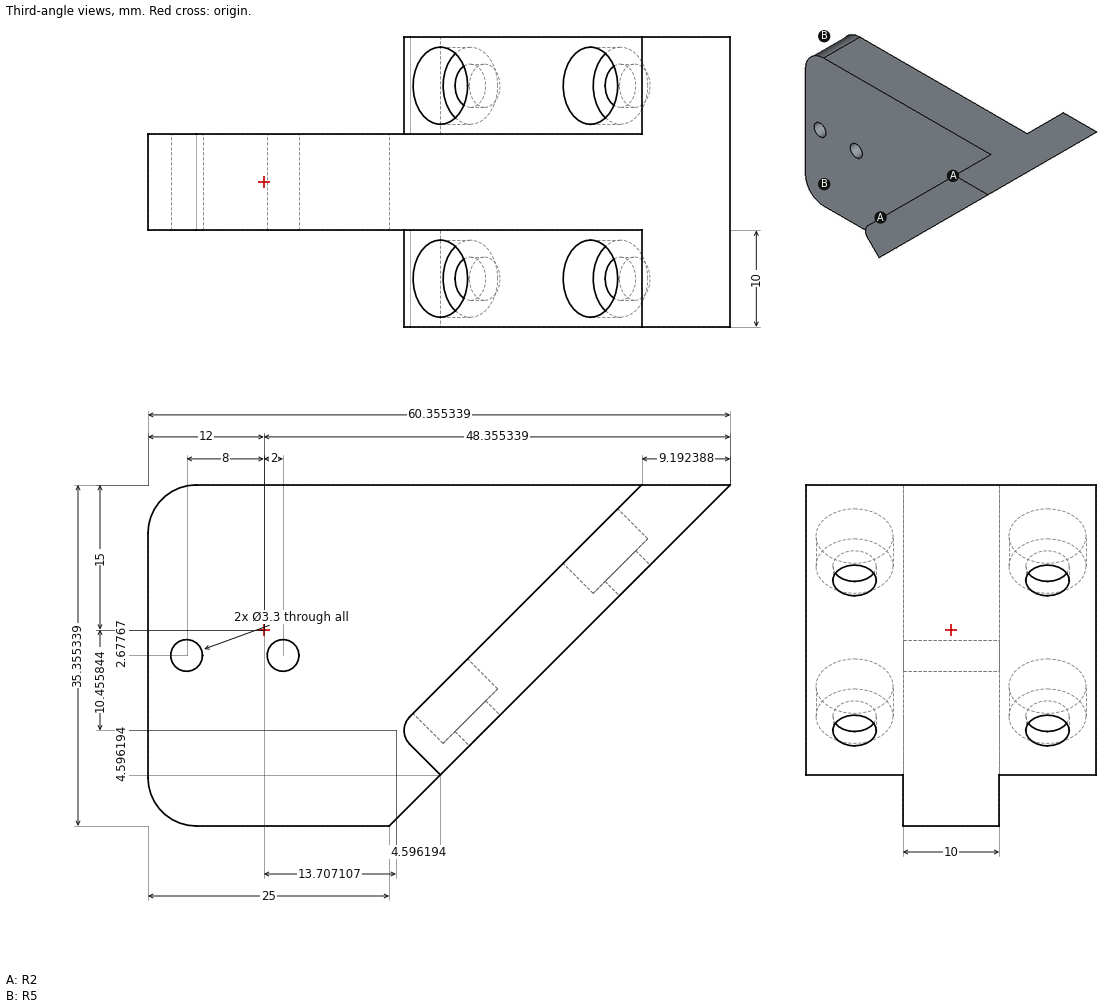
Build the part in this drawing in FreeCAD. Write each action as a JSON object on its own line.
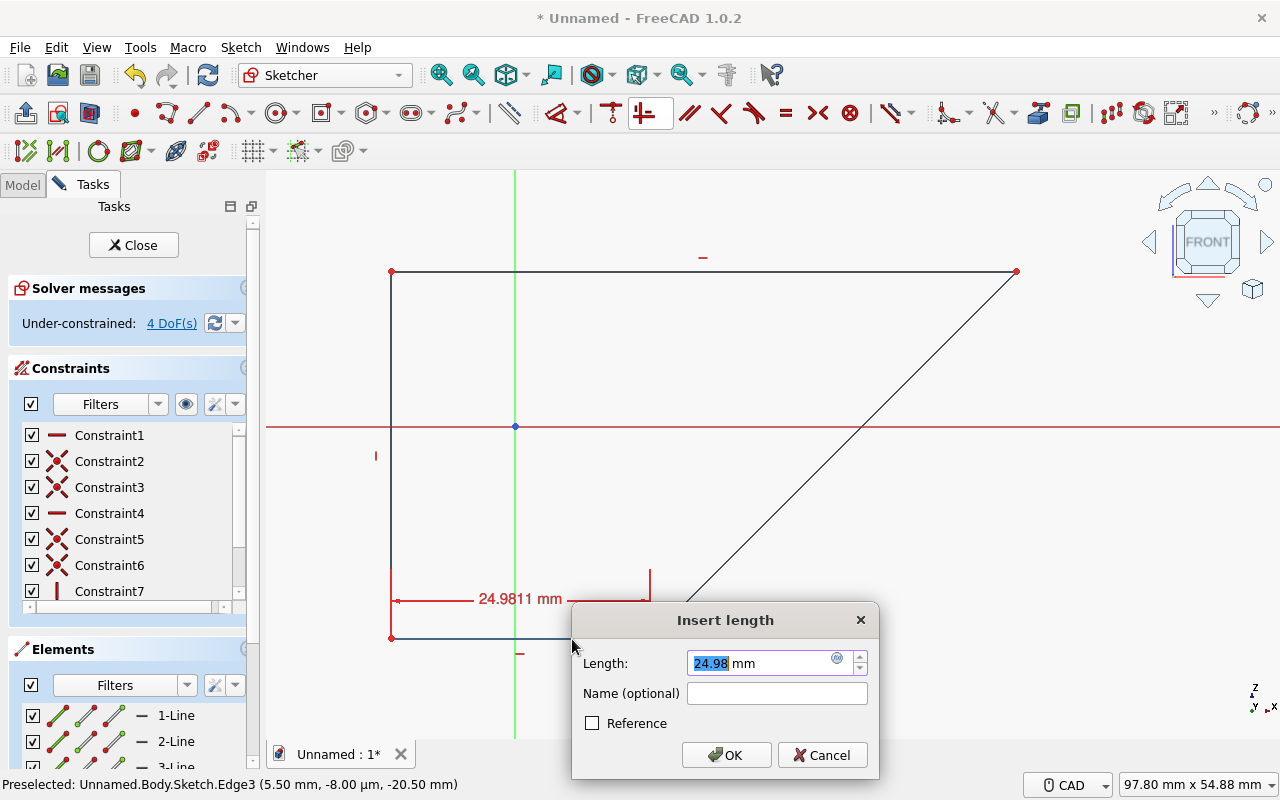
{"action": "type", "text": "25"}
{"action": "key", "text": "Return"}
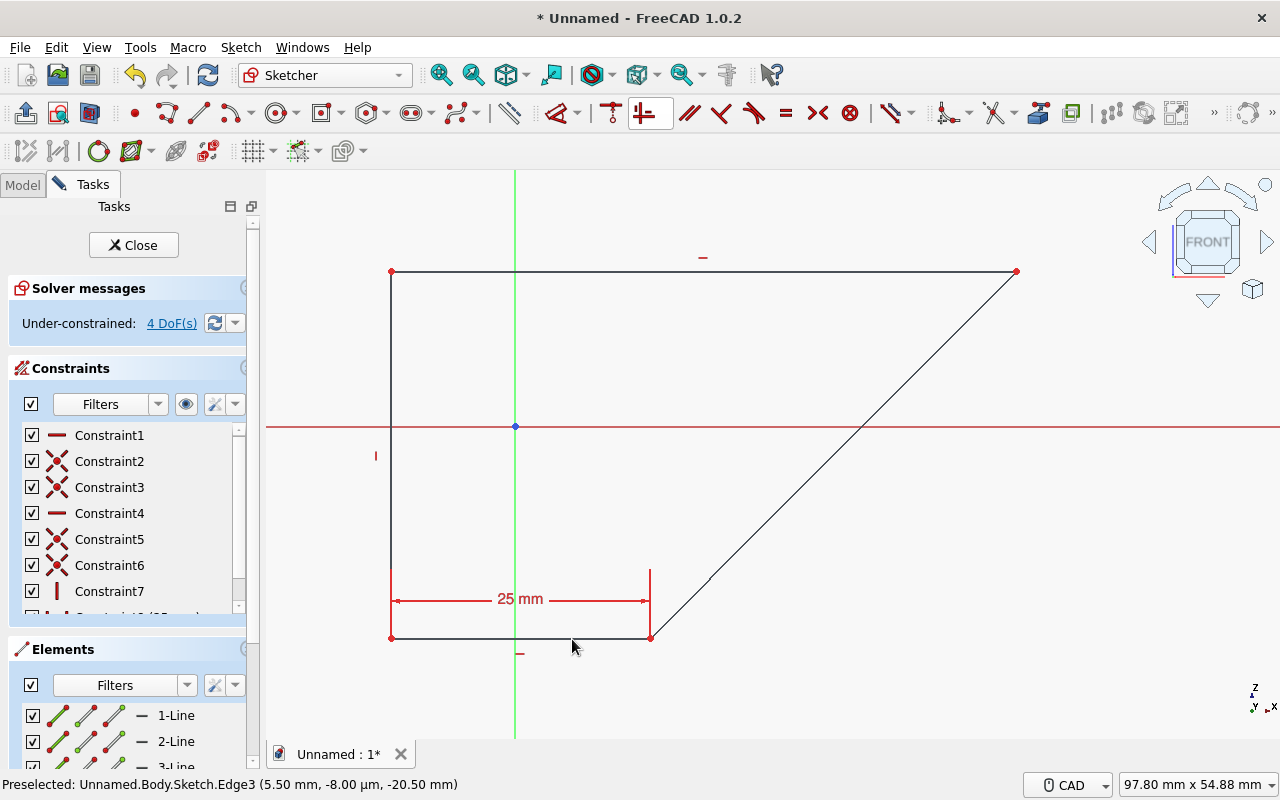
{"action": "left_click", "coordinate": [391, 272]}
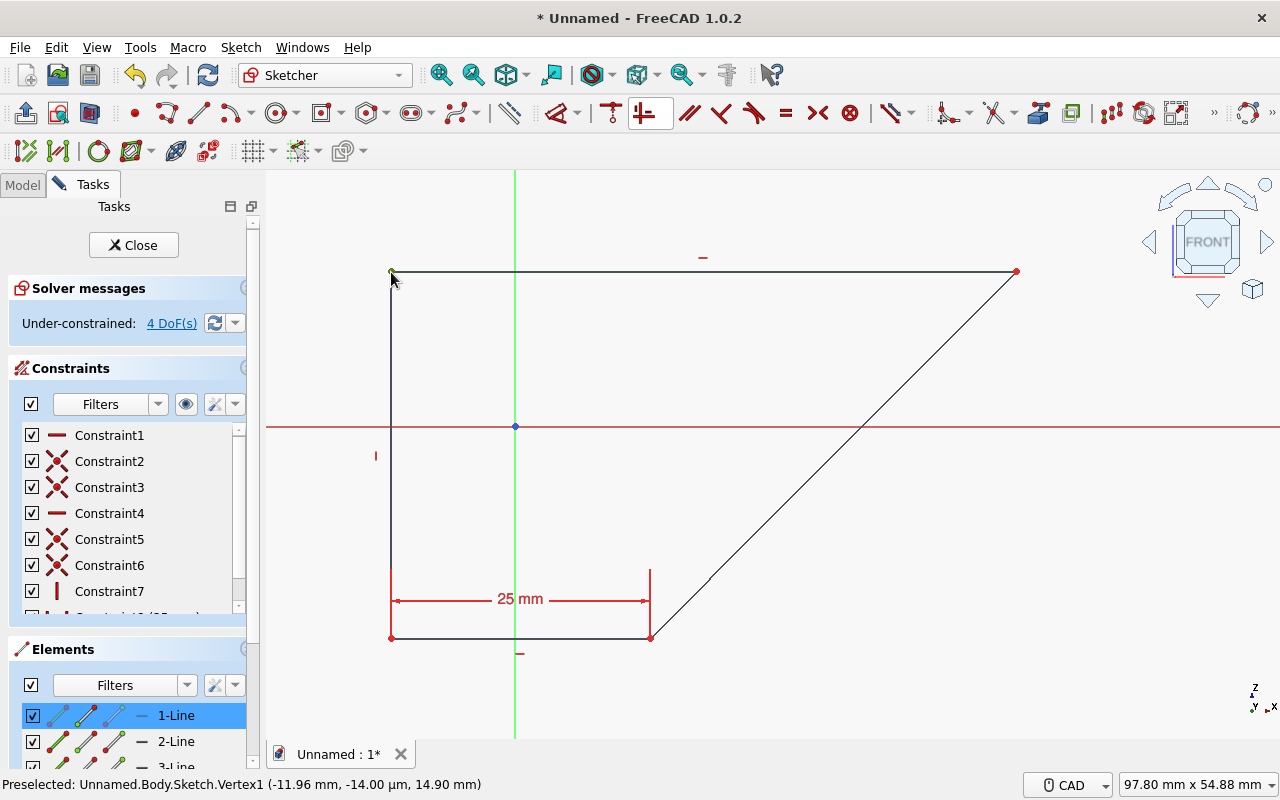
{"action": "left_click", "coordinate": [580, 114]}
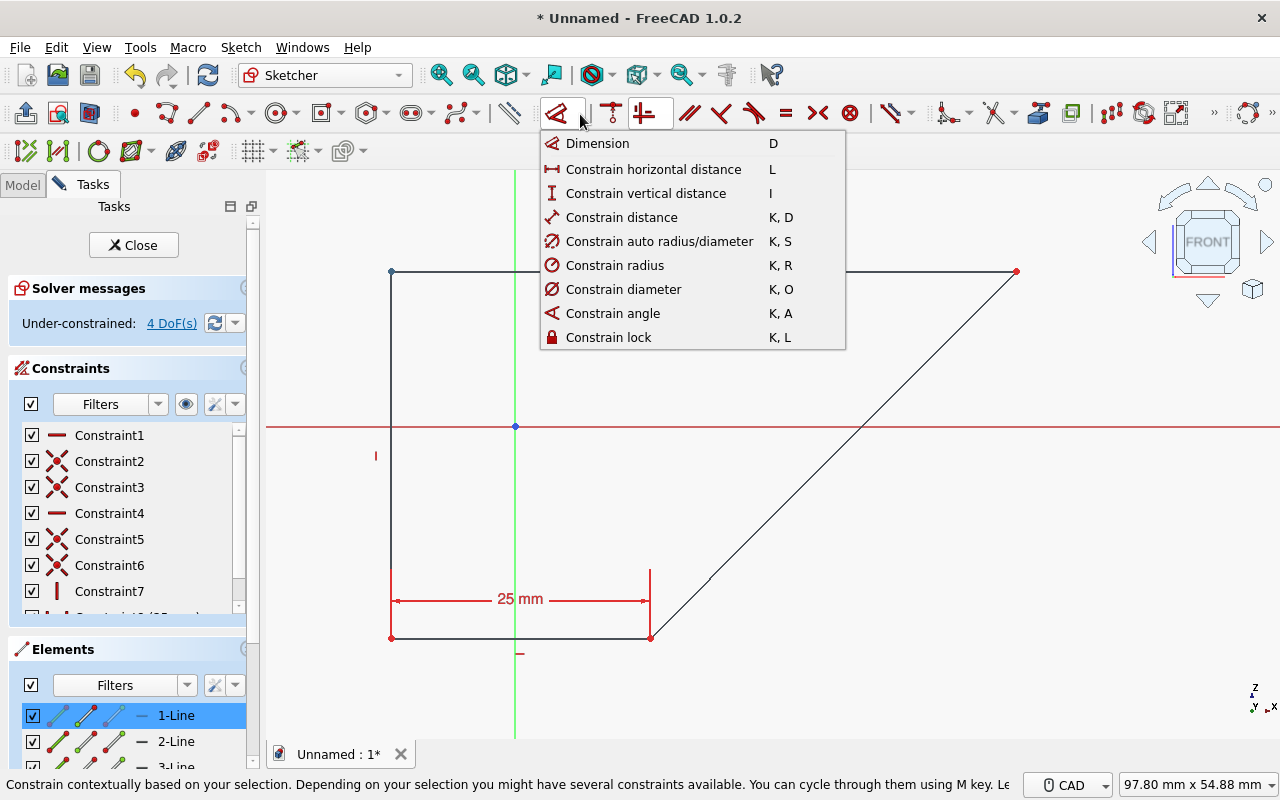
{"action": "left_click", "coordinate": [693, 169]}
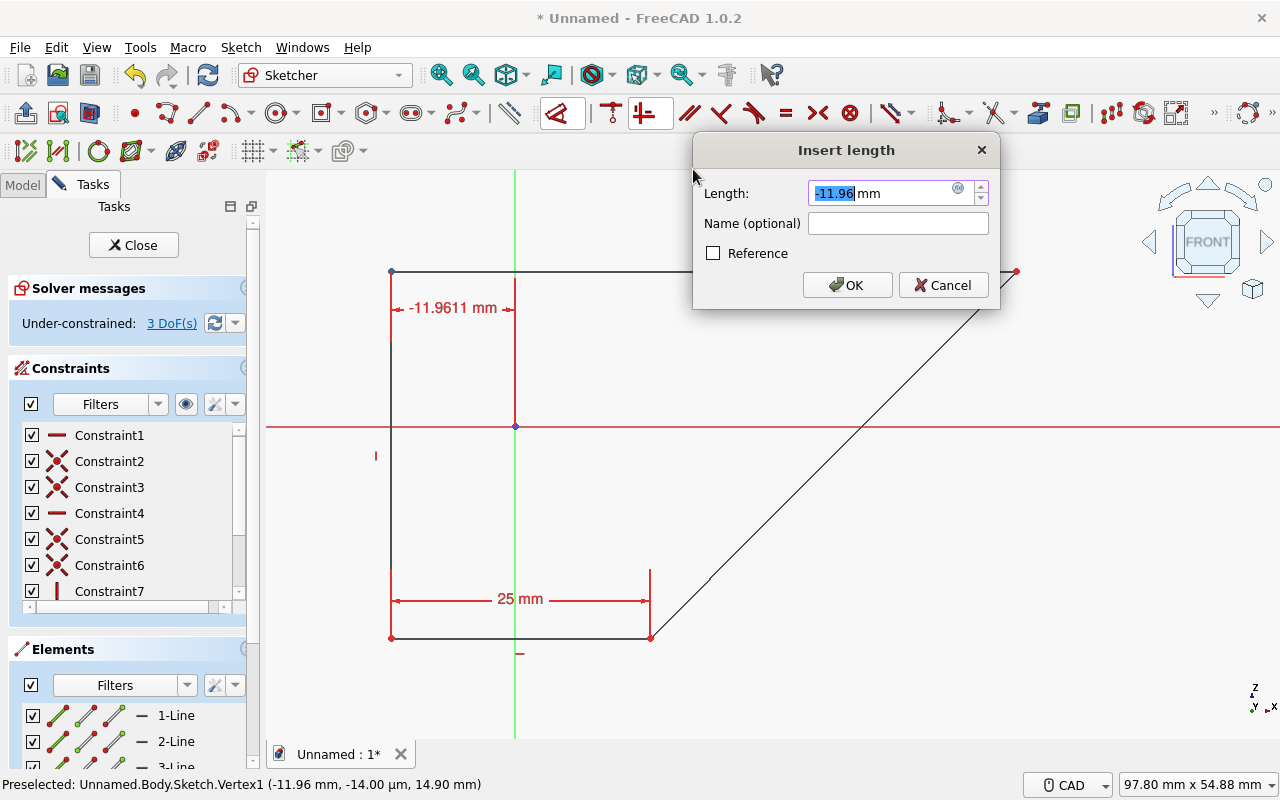
{"action": "type", "text": "-12"}
{"action": "key", "text": "Return"}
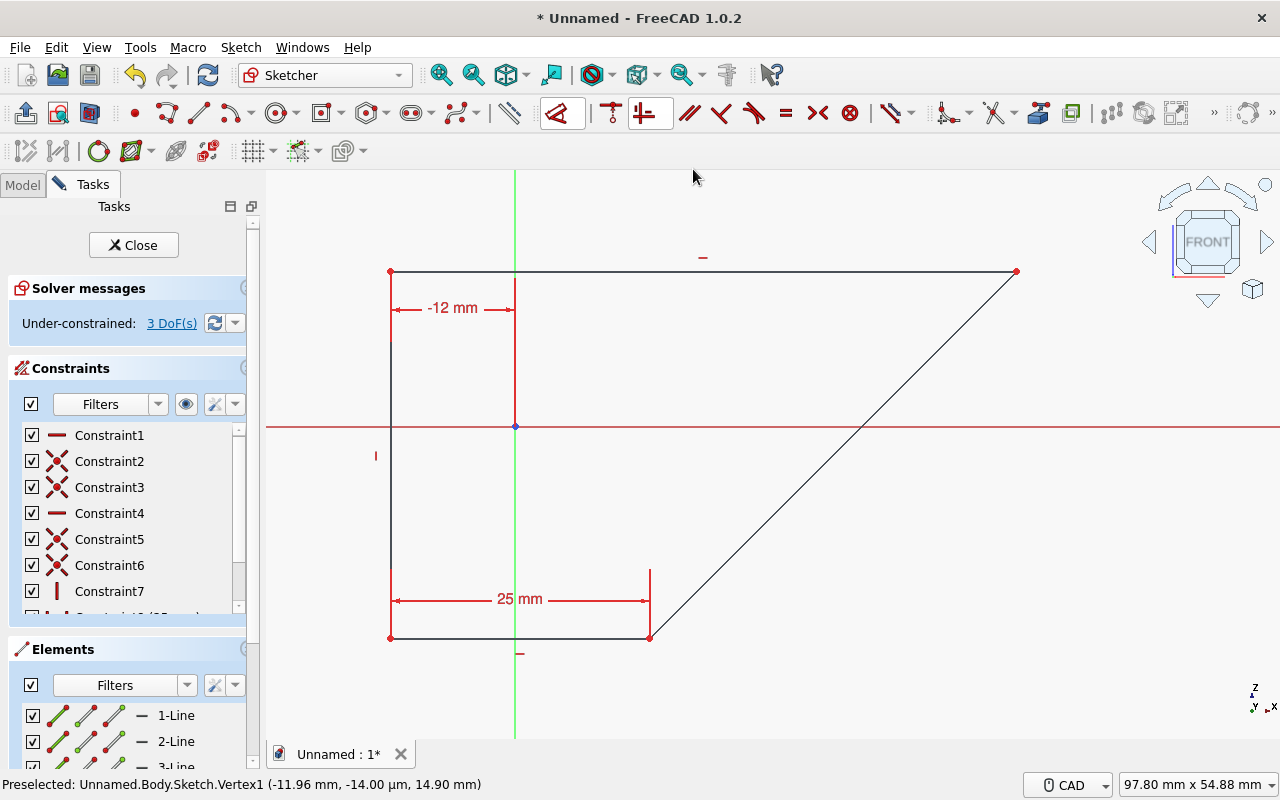
{"action": "left_click", "coordinate": [391, 272]}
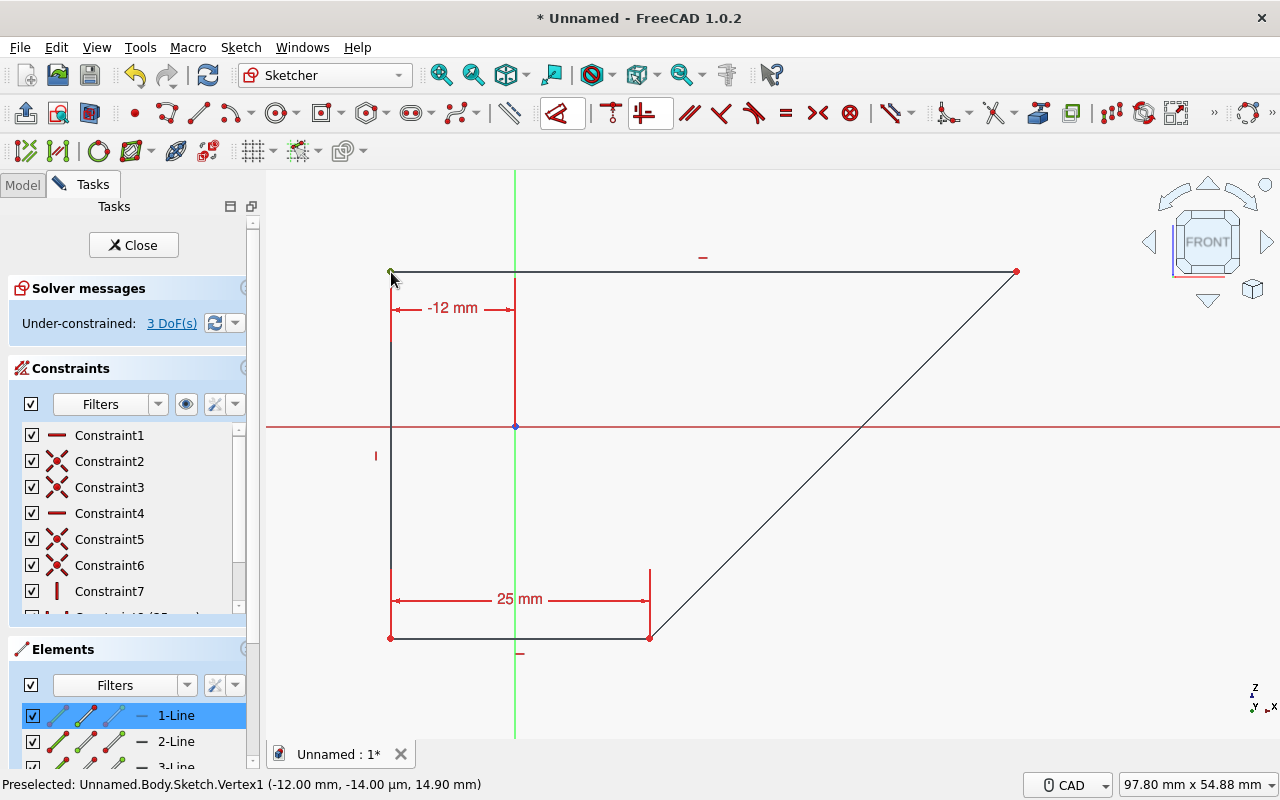
{"action": "key", "text": "i"}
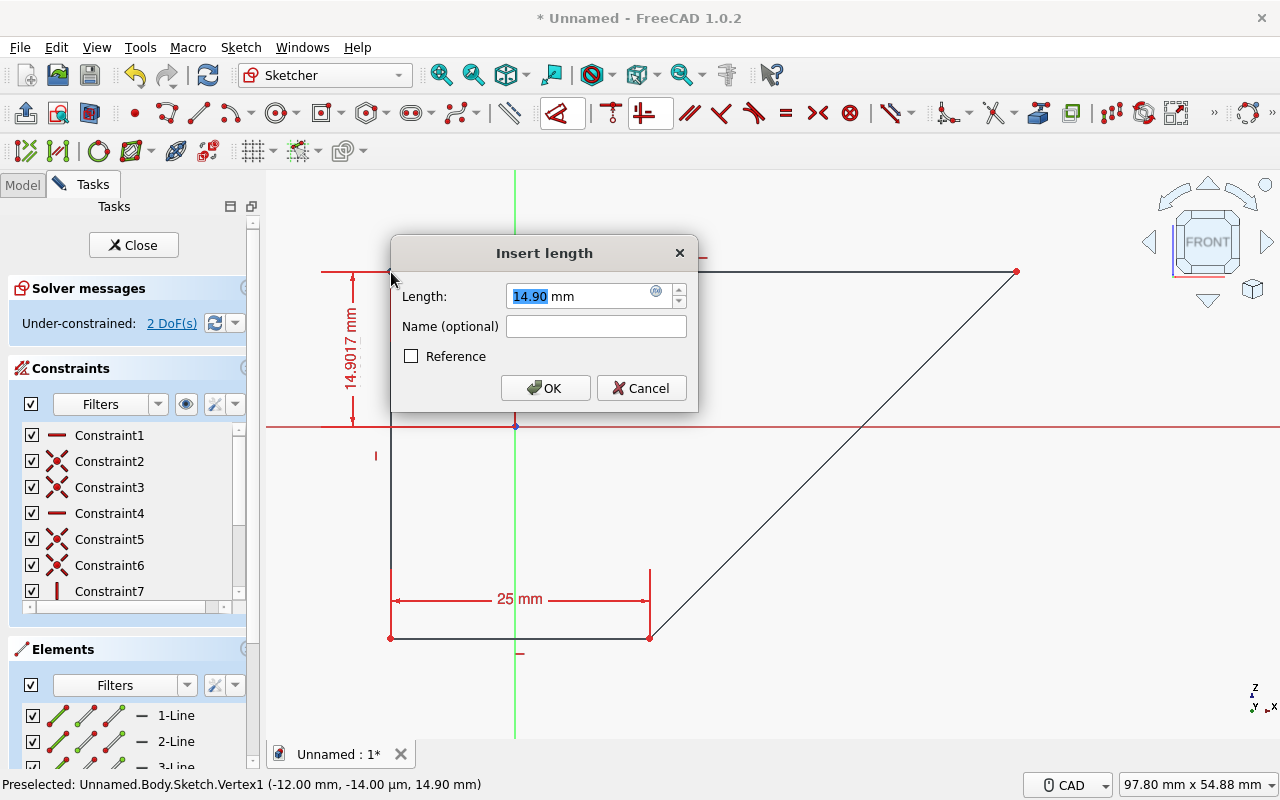
{"action": "type", "text": "15"}
{"action": "key", "text": "Return"}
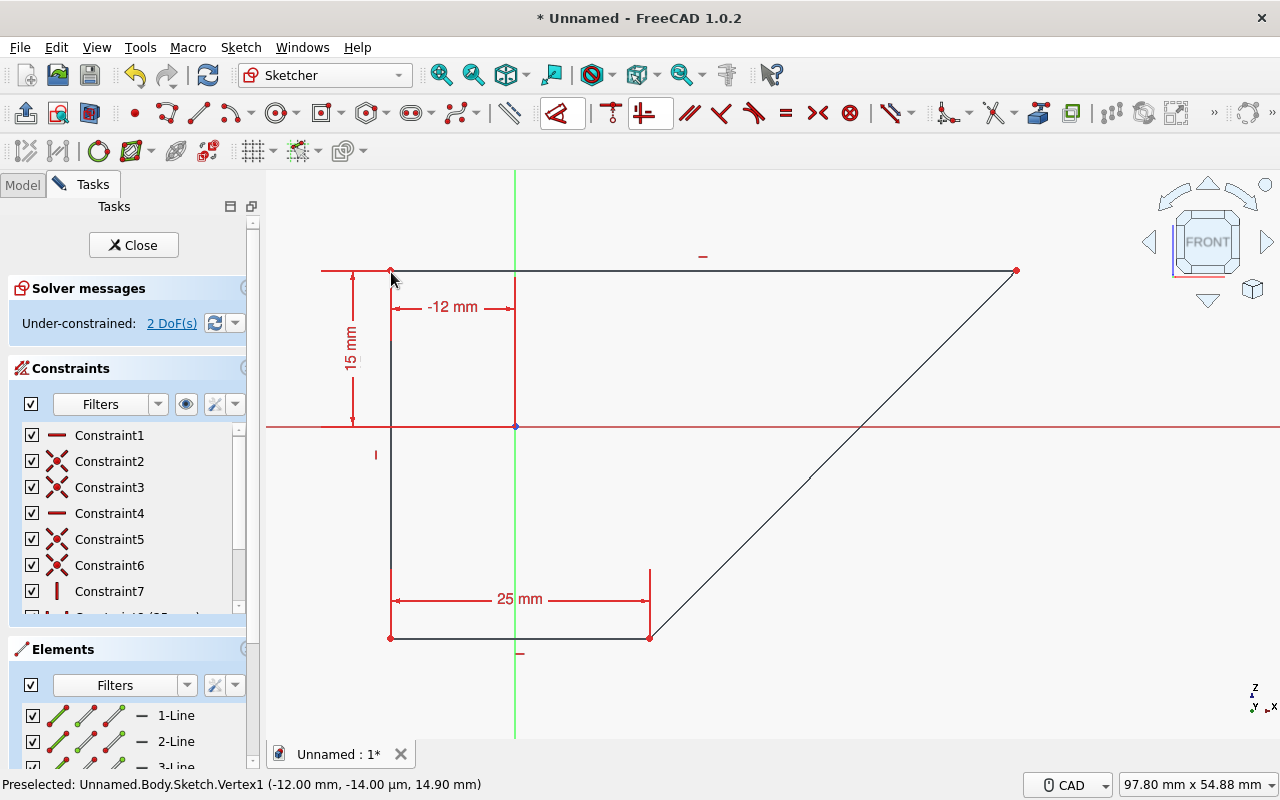
{"action": "left_click", "coordinate": [578, 271]}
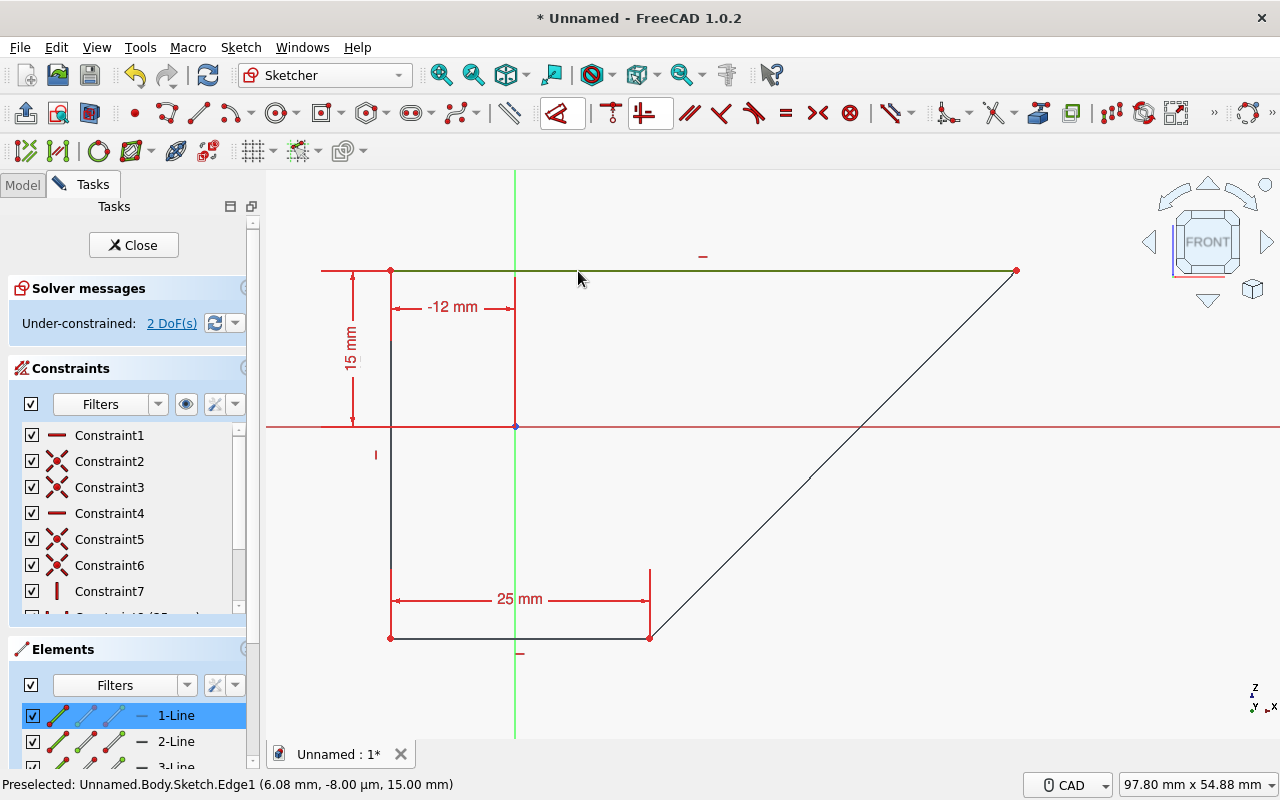
{"action": "key", "text": "l"}